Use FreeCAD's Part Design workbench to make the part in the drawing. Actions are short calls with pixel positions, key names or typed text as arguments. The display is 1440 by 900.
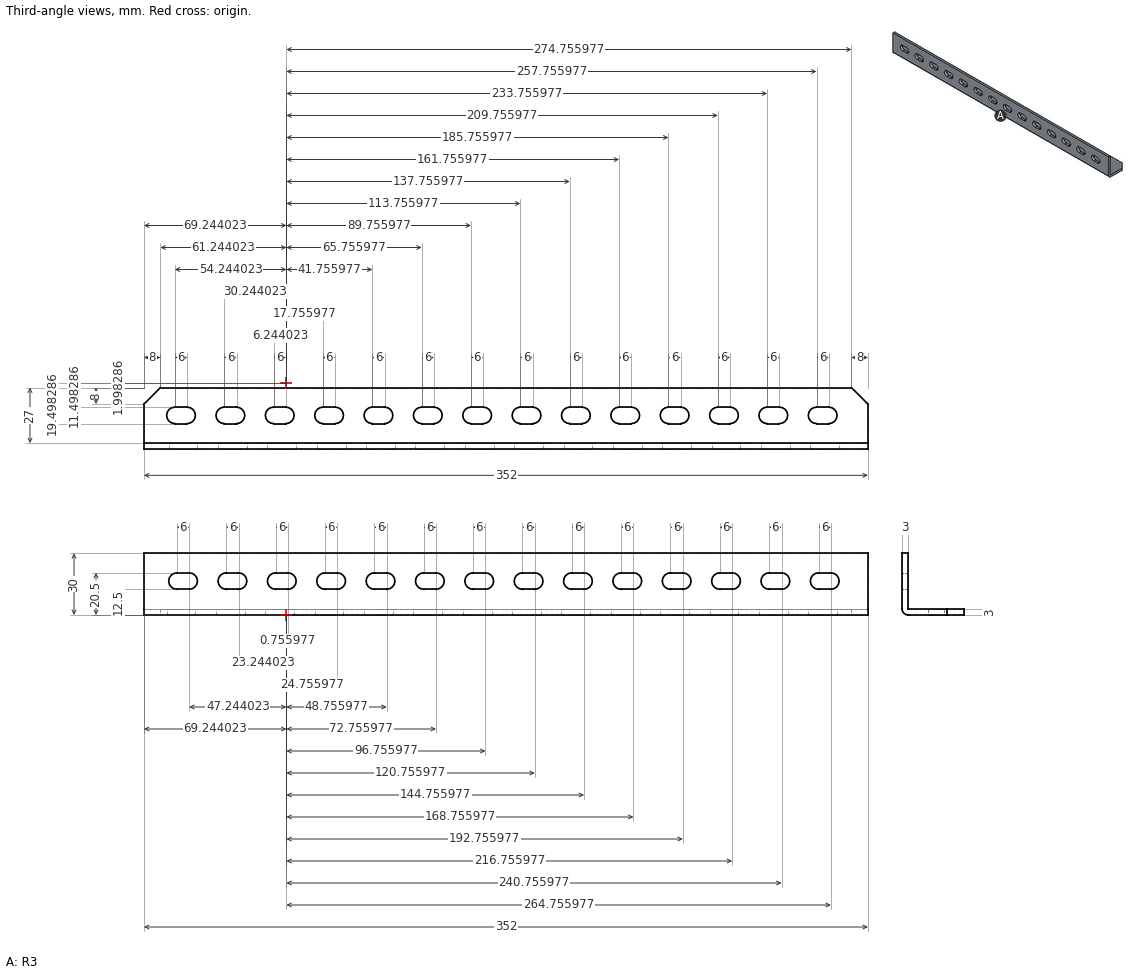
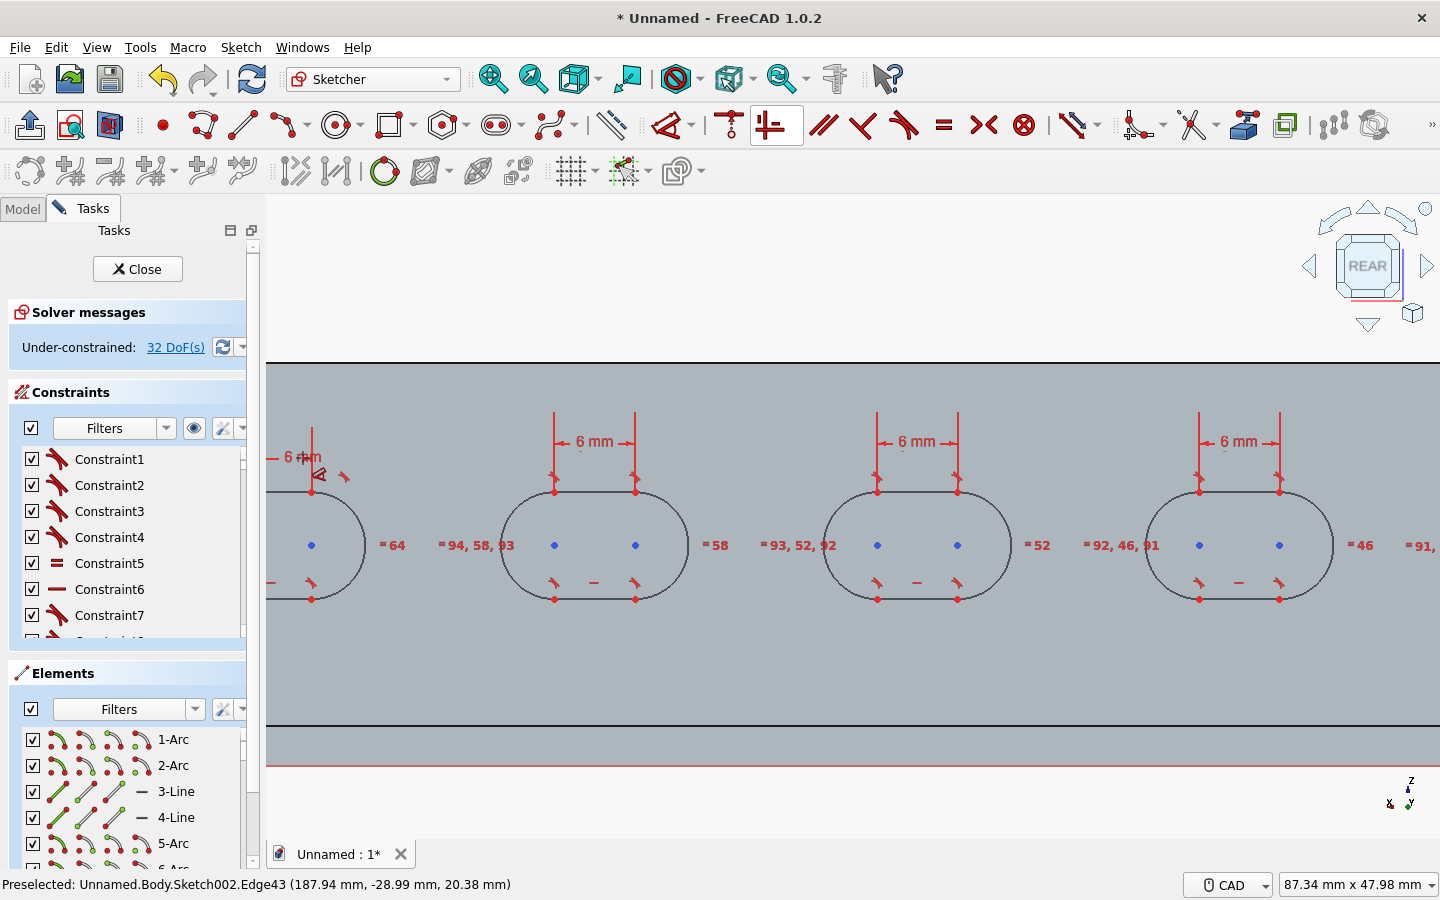
scroll(662, 494, down, 9)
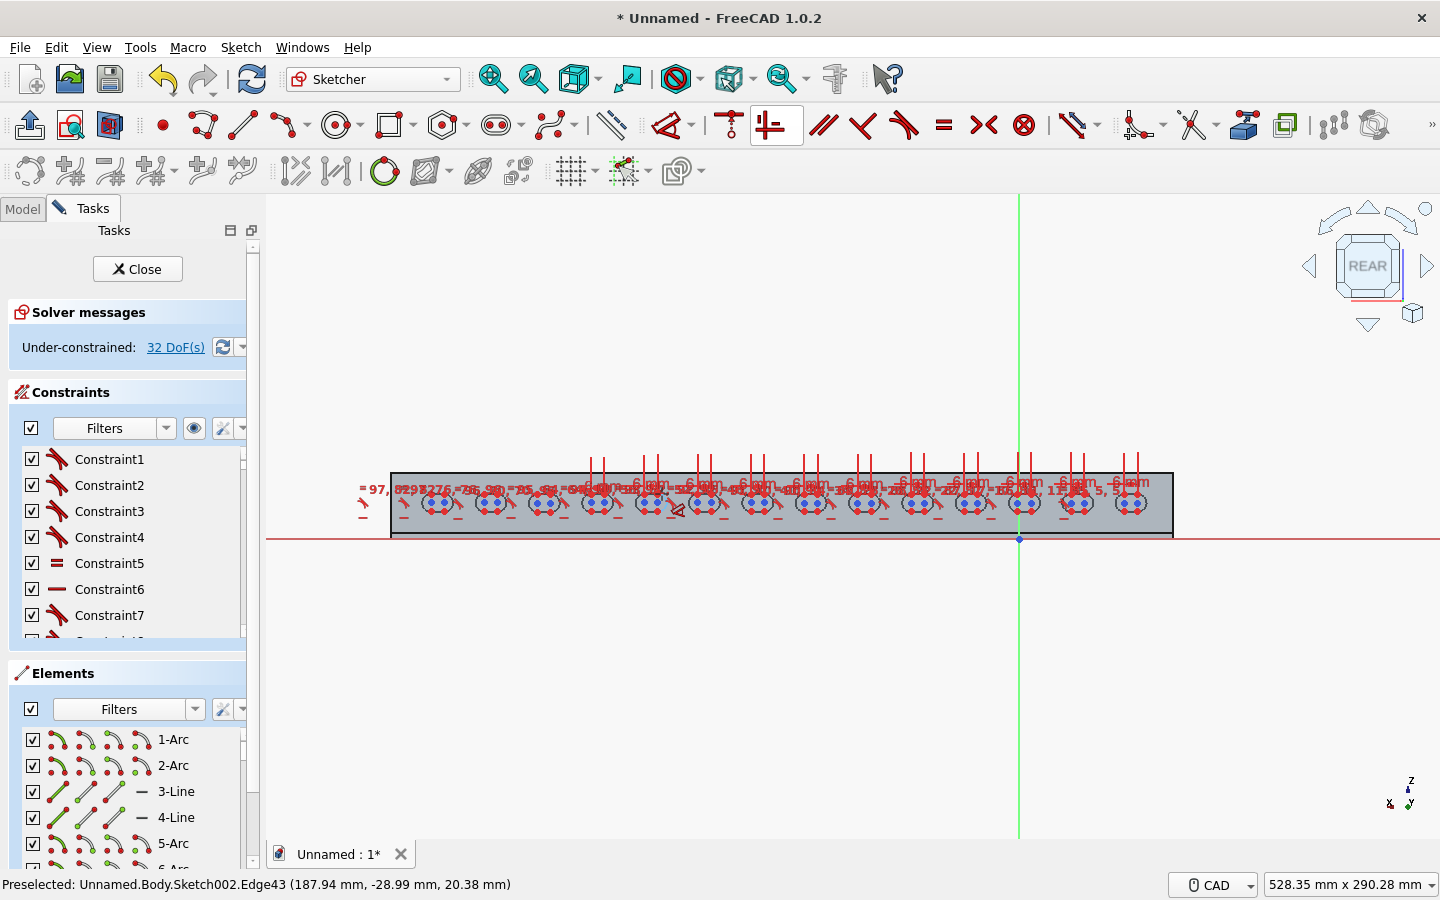
scroll(542, 494, up, 7)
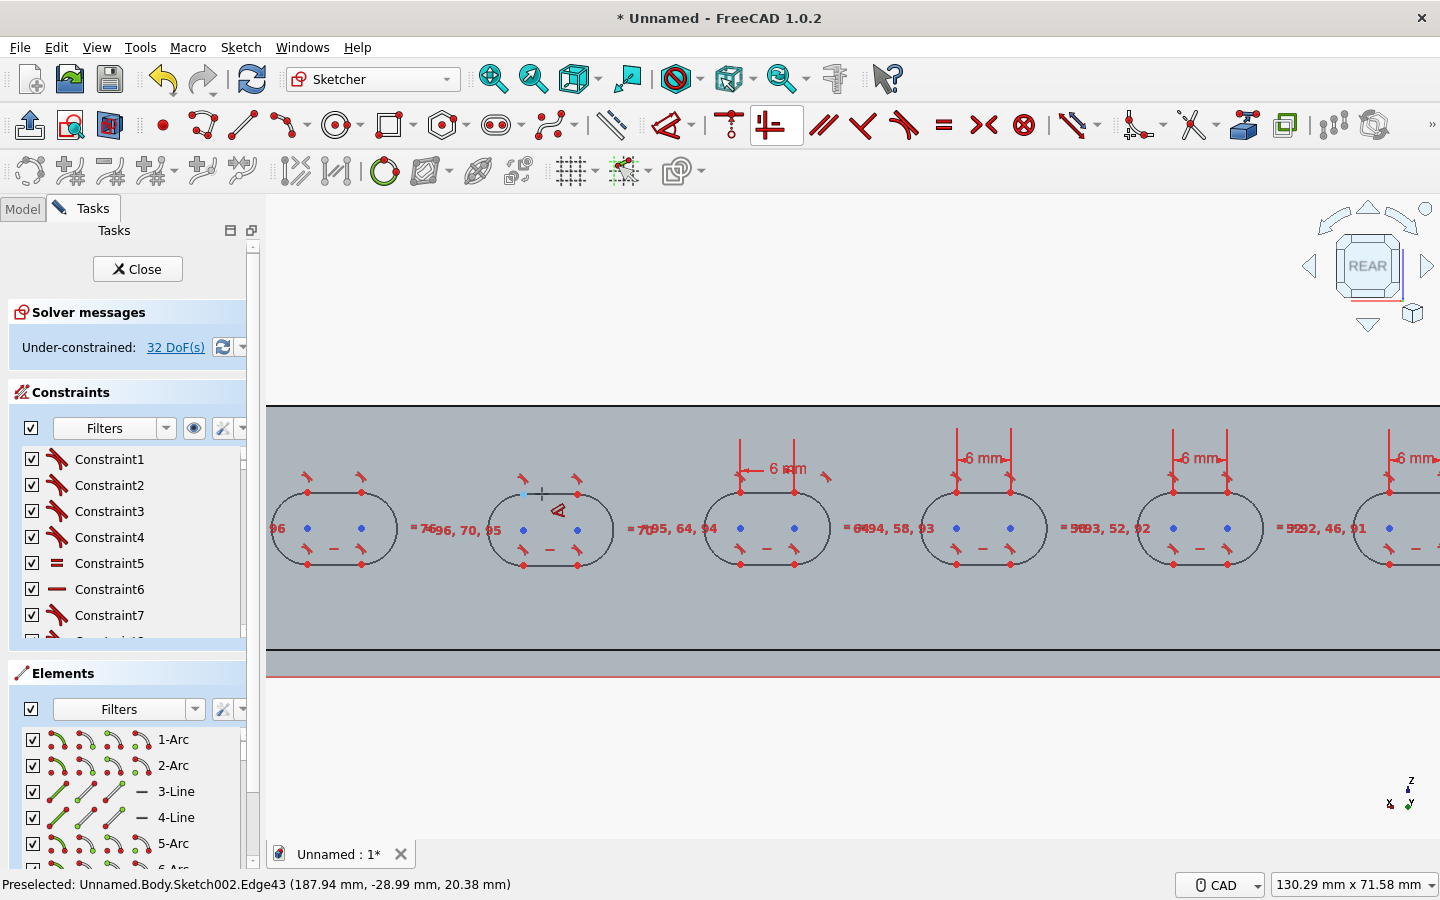
click(540, 494)
click(551, 460)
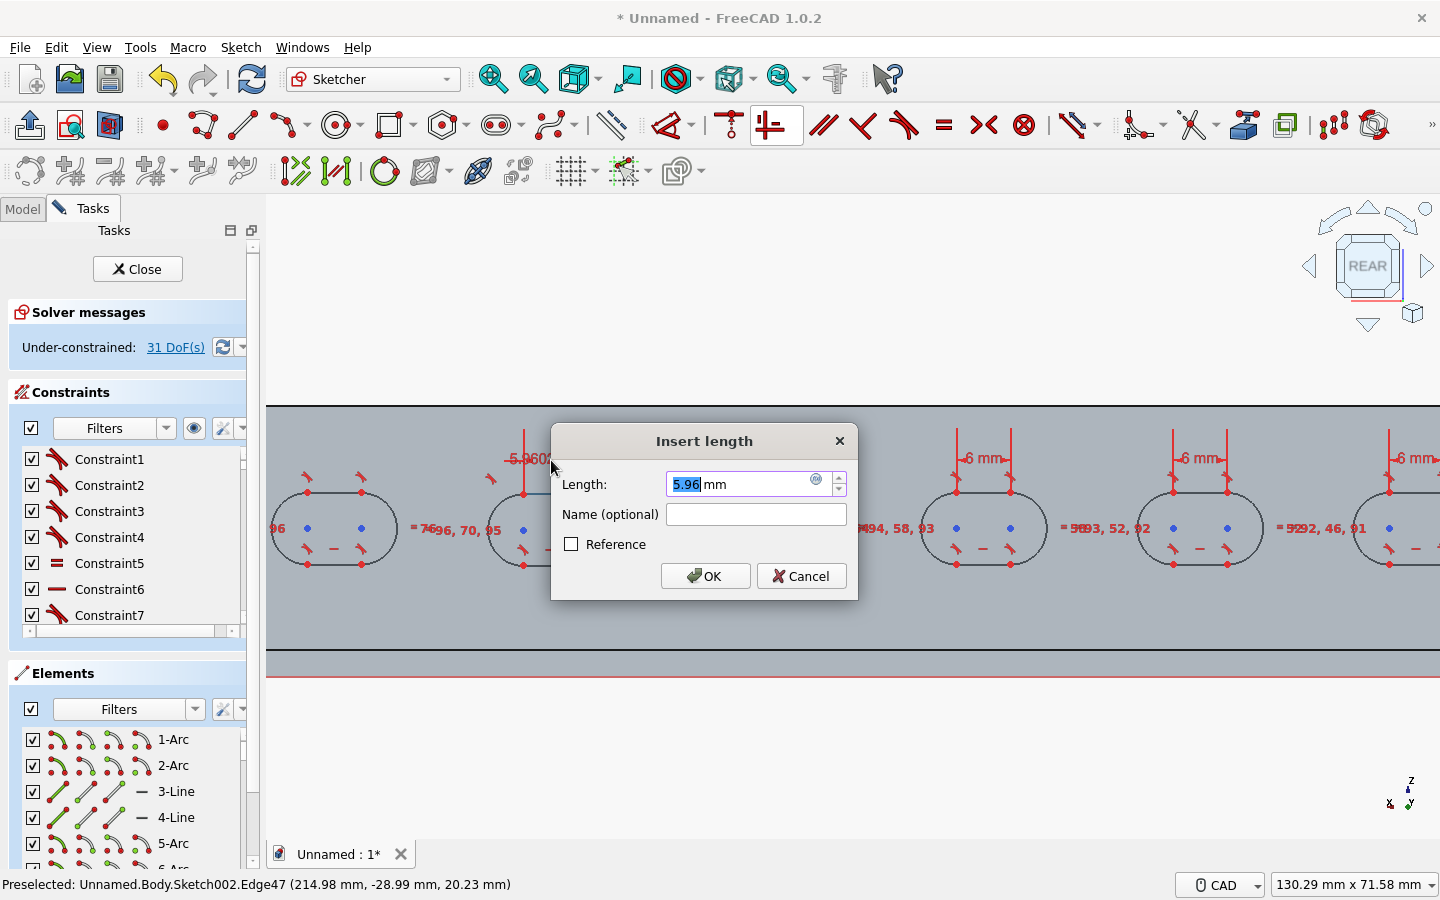
text(6)
key(Return)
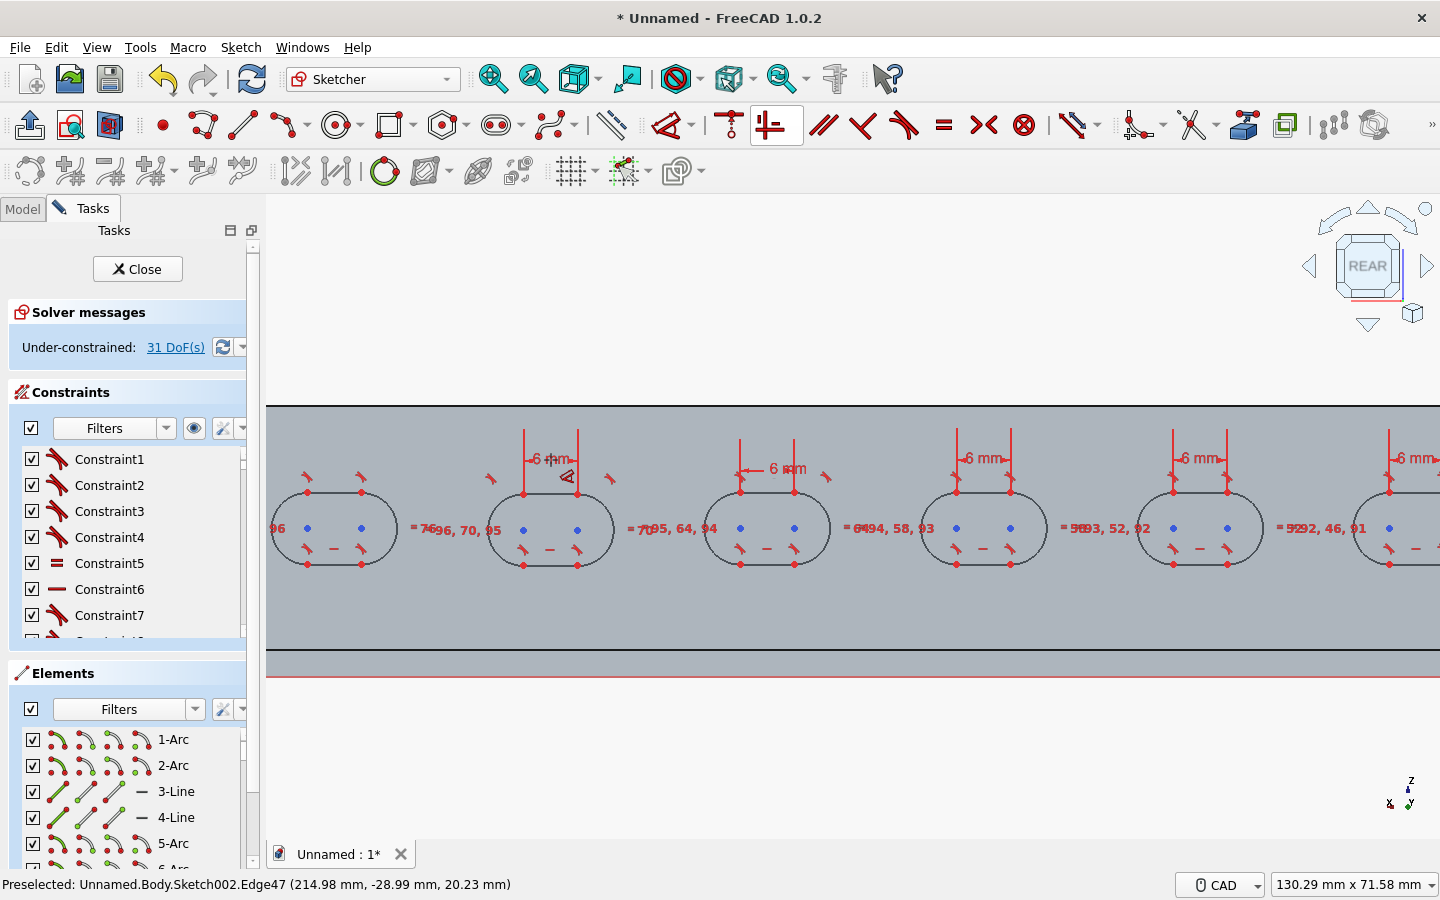
click(324, 493)
click(334, 459)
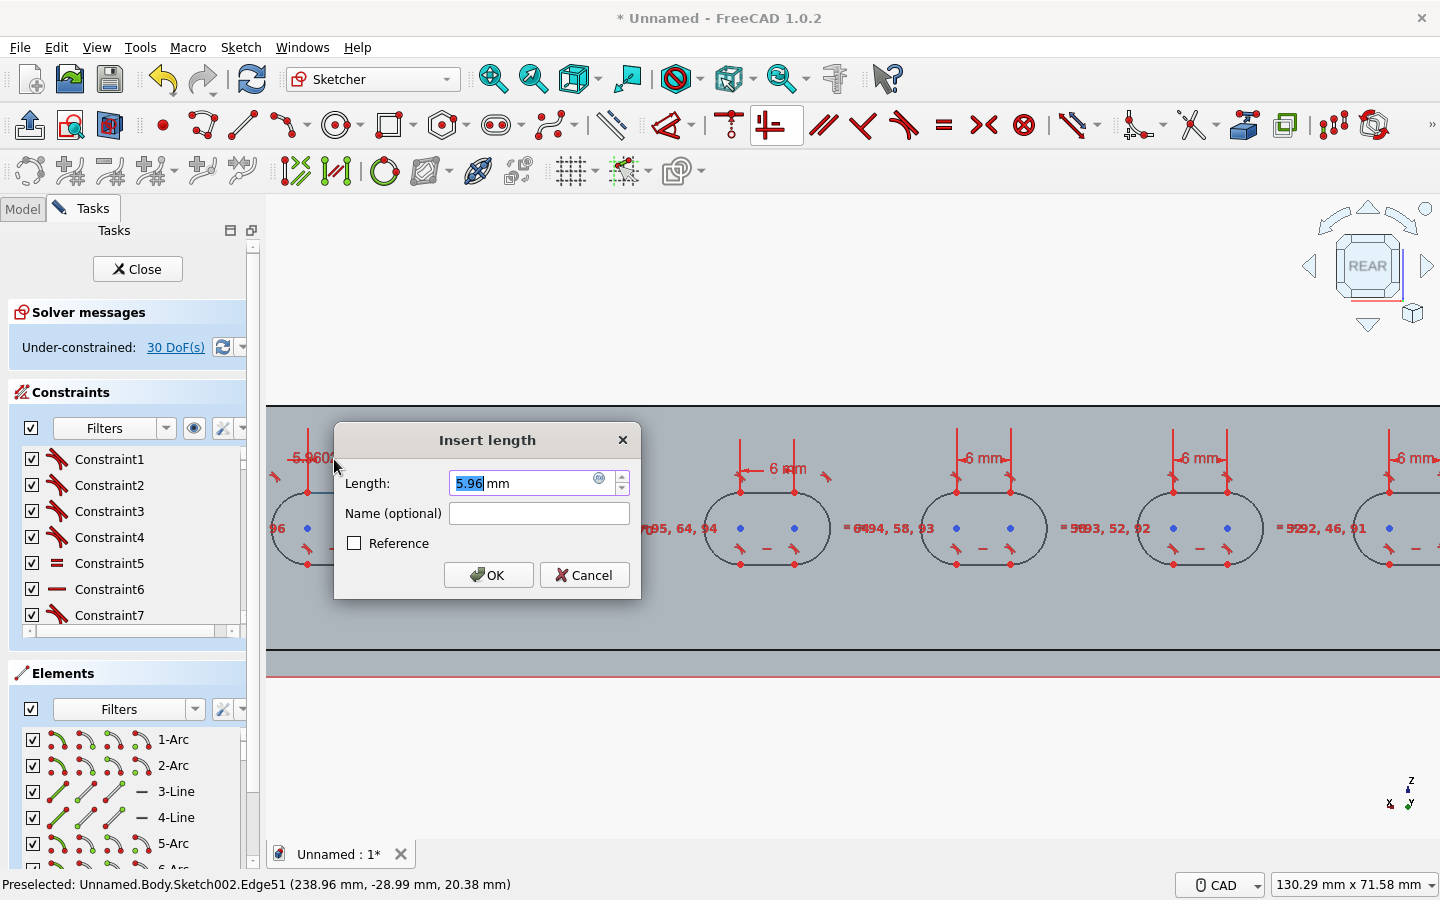
text(6)
key(Return)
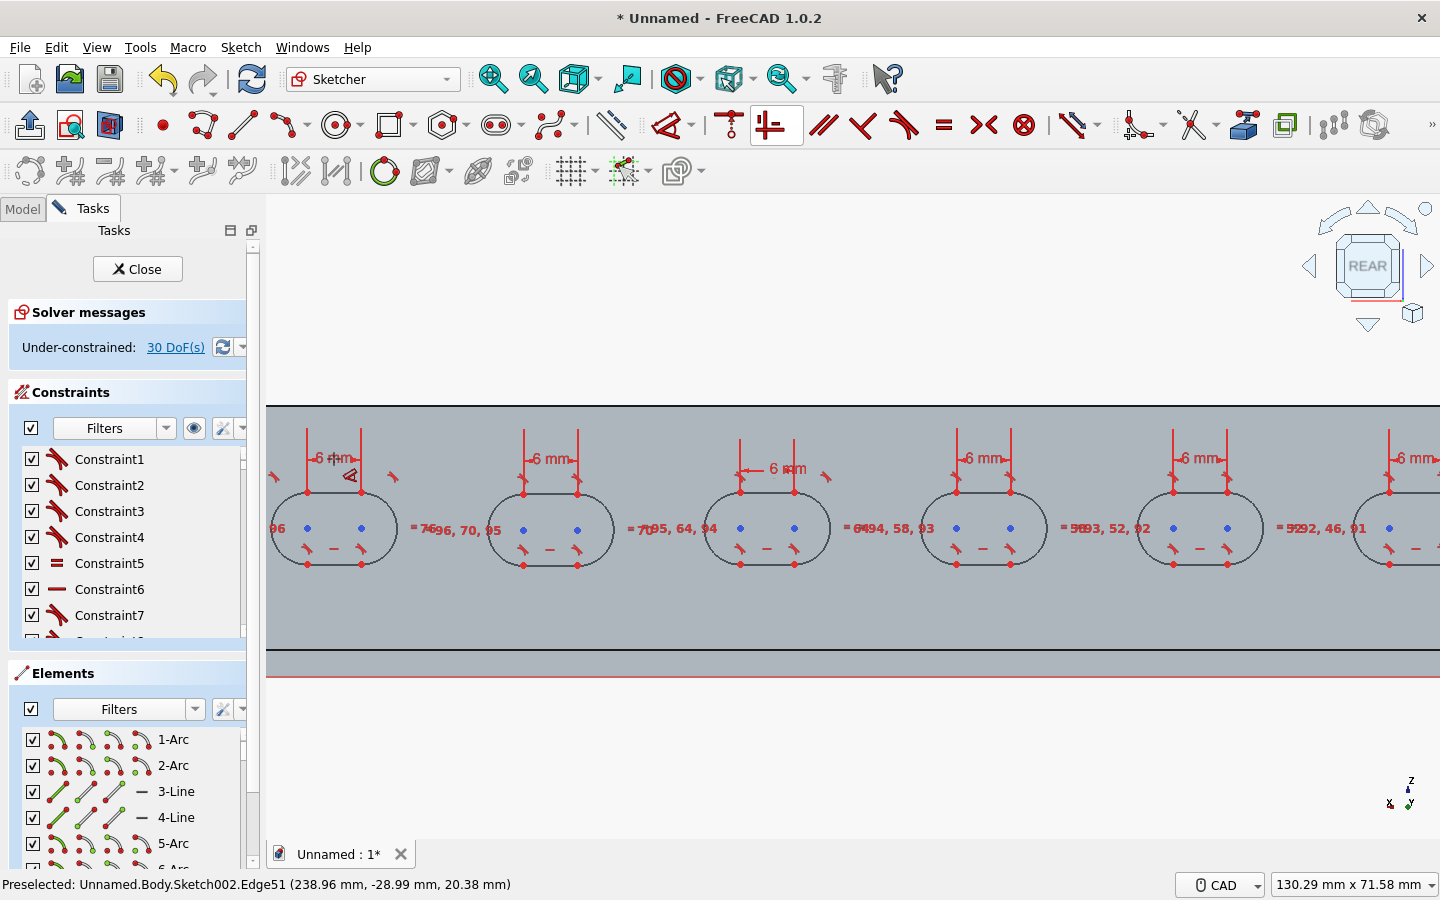
scroll(542, 494, down, 7)